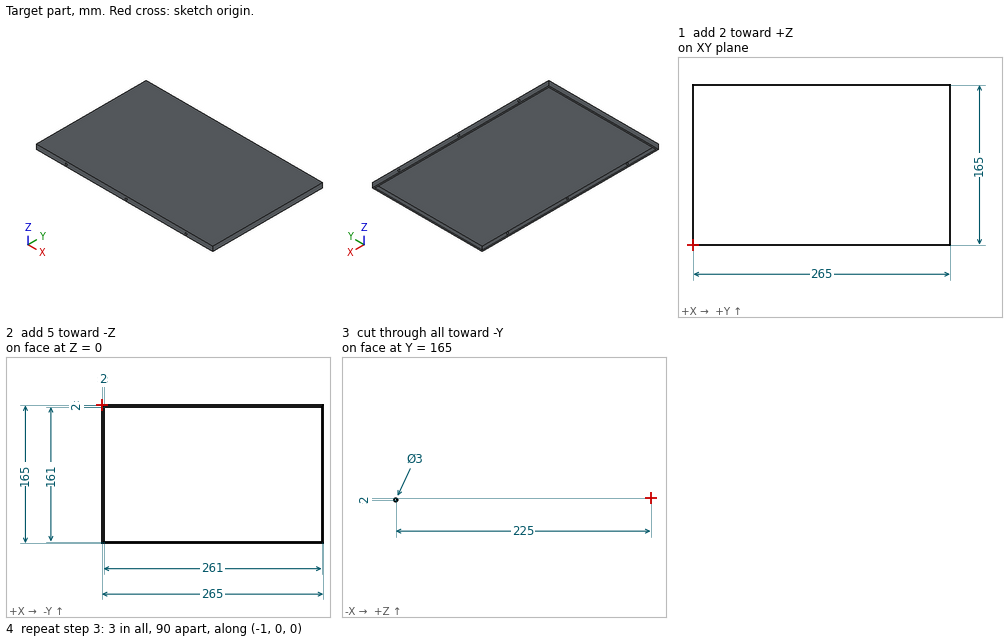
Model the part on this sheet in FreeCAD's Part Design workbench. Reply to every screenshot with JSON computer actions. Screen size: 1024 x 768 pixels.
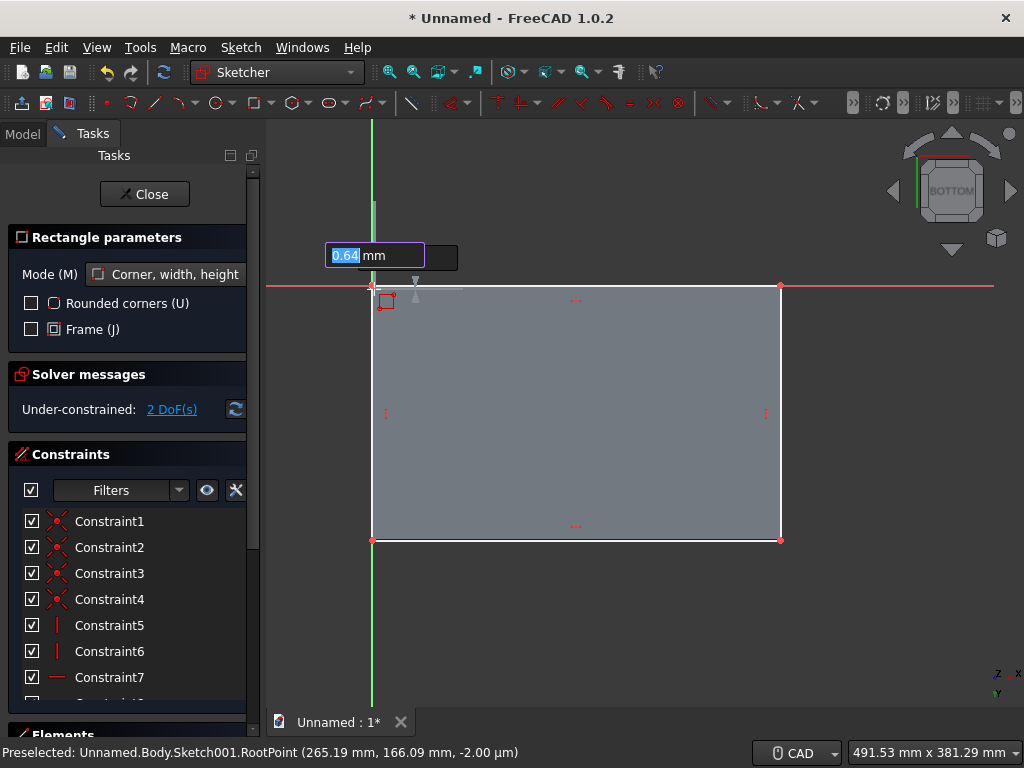
{"action": "scroll", "coordinate": [778, 537], "scroll_direction": "up", "scroll_amount": 9}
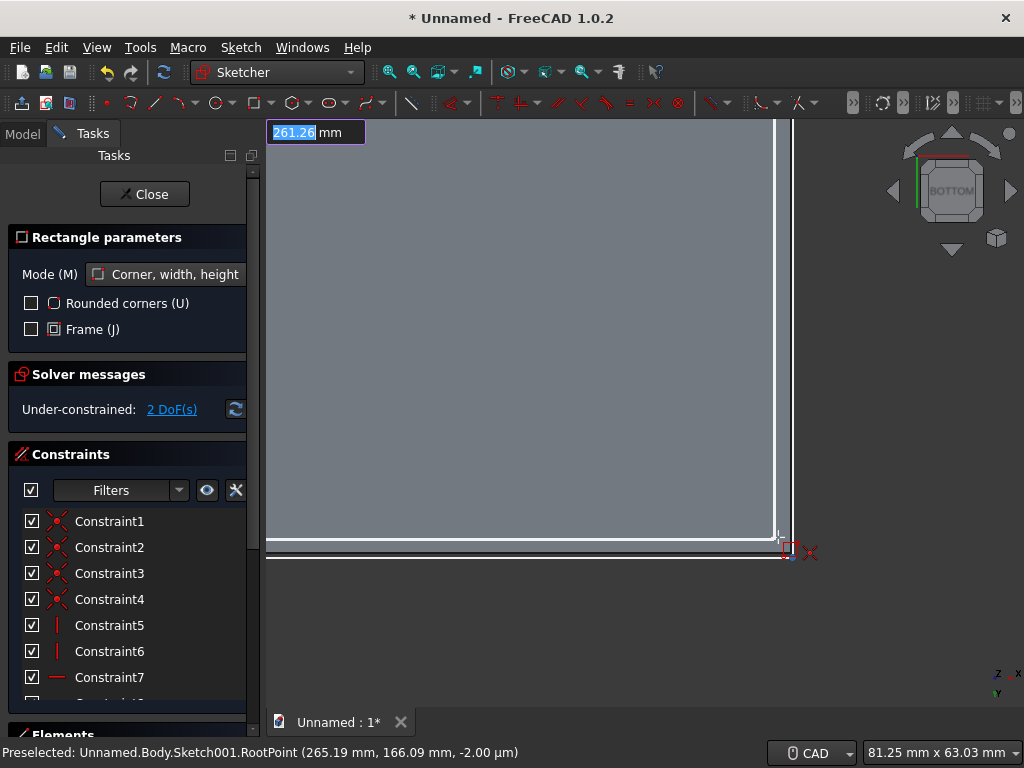
{"action": "left_click", "coordinate": [772, 535]}
{"action": "key", "text": "Escape"}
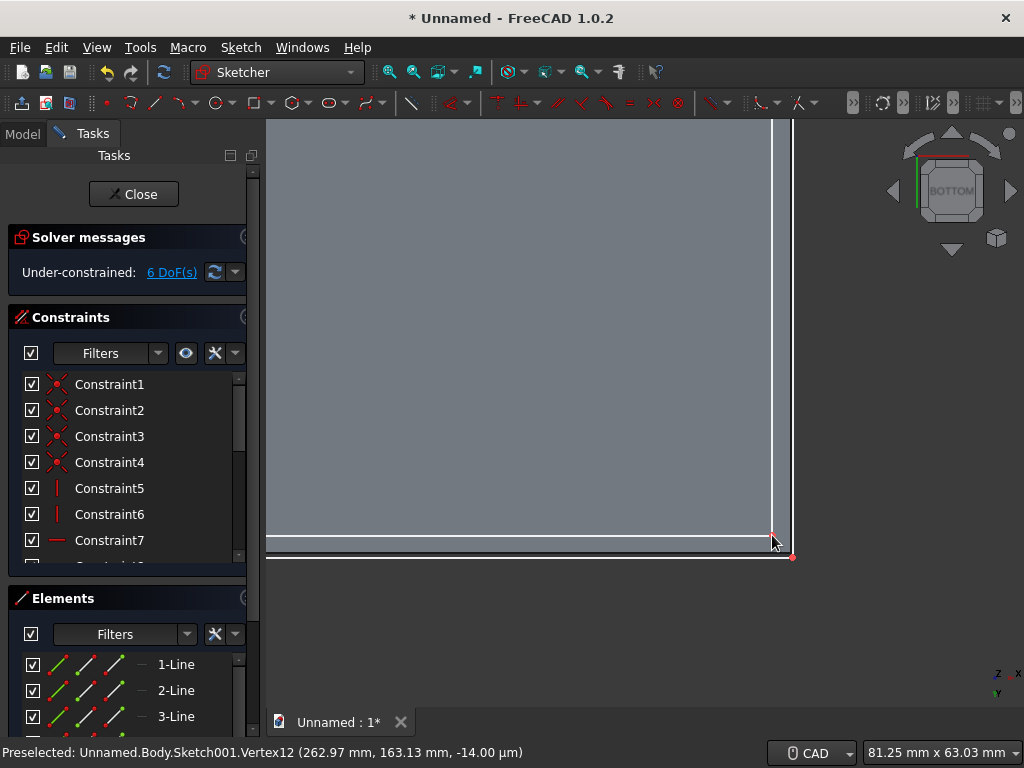
{"action": "left_click", "coordinate": [450, 104]}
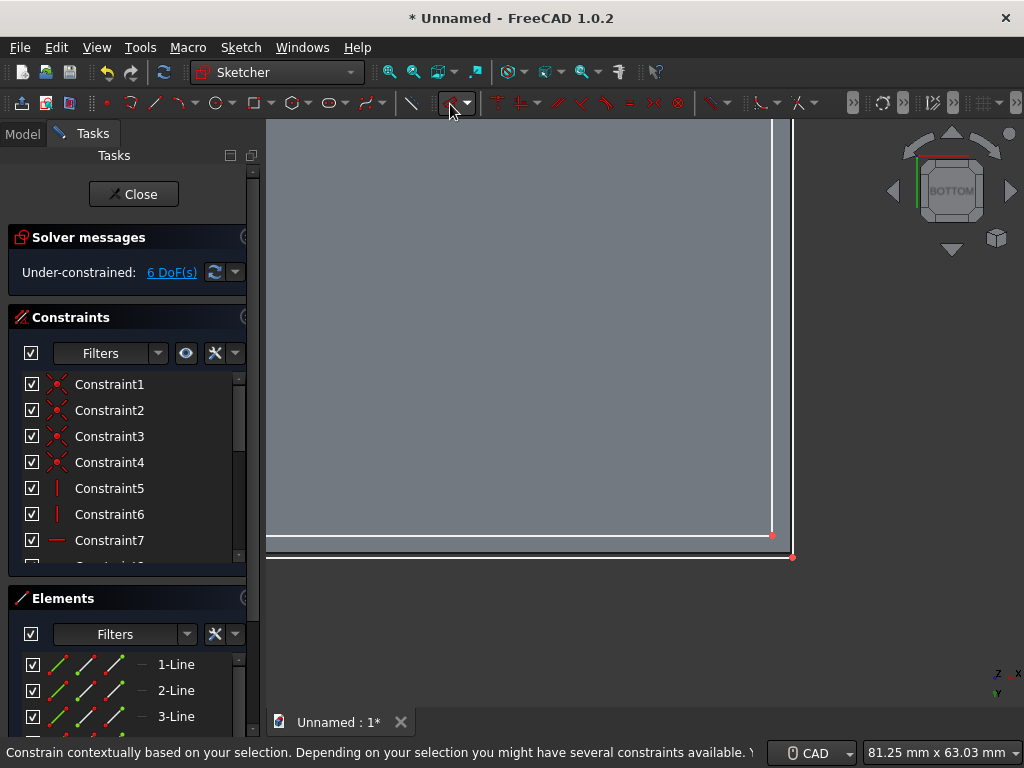
{"action": "scroll", "coordinate": [779, 538], "scroll_direction": "down", "scroll_amount": 9}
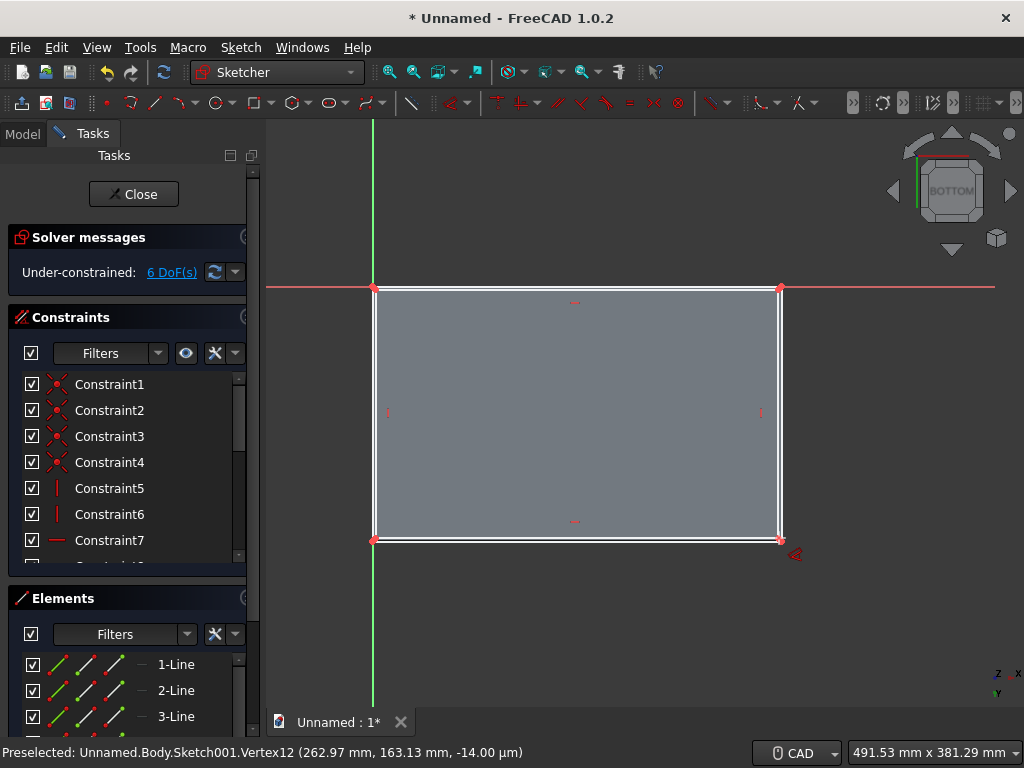
{"action": "scroll", "coordinate": [376, 290], "scroll_direction": "up", "scroll_amount": 13}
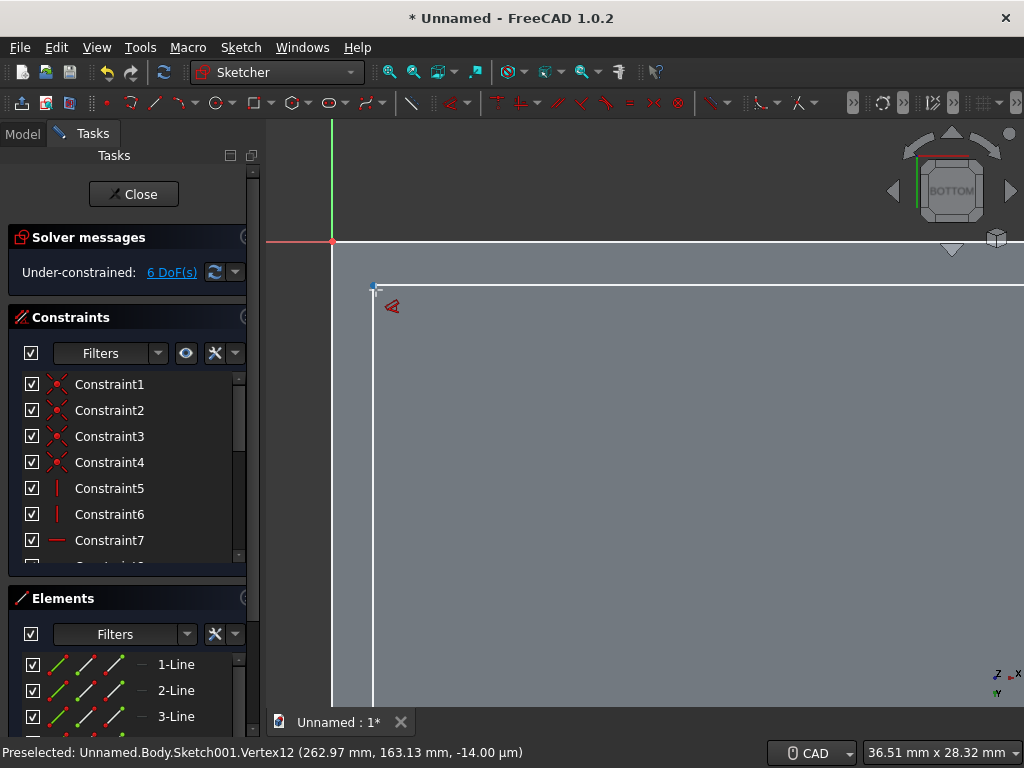
{"action": "left_click", "coordinate": [373, 285]}
{"action": "left_click", "coordinate": [353, 208]}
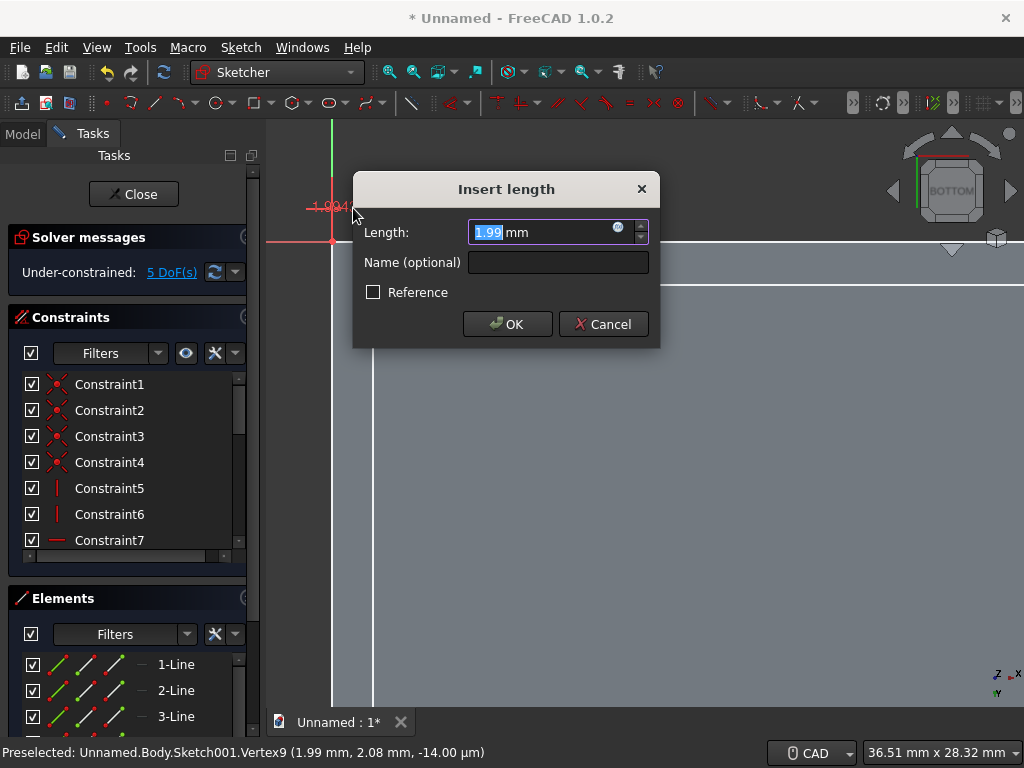
{"action": "type", "text": "2"}
{"action": "key", "text": "Return"}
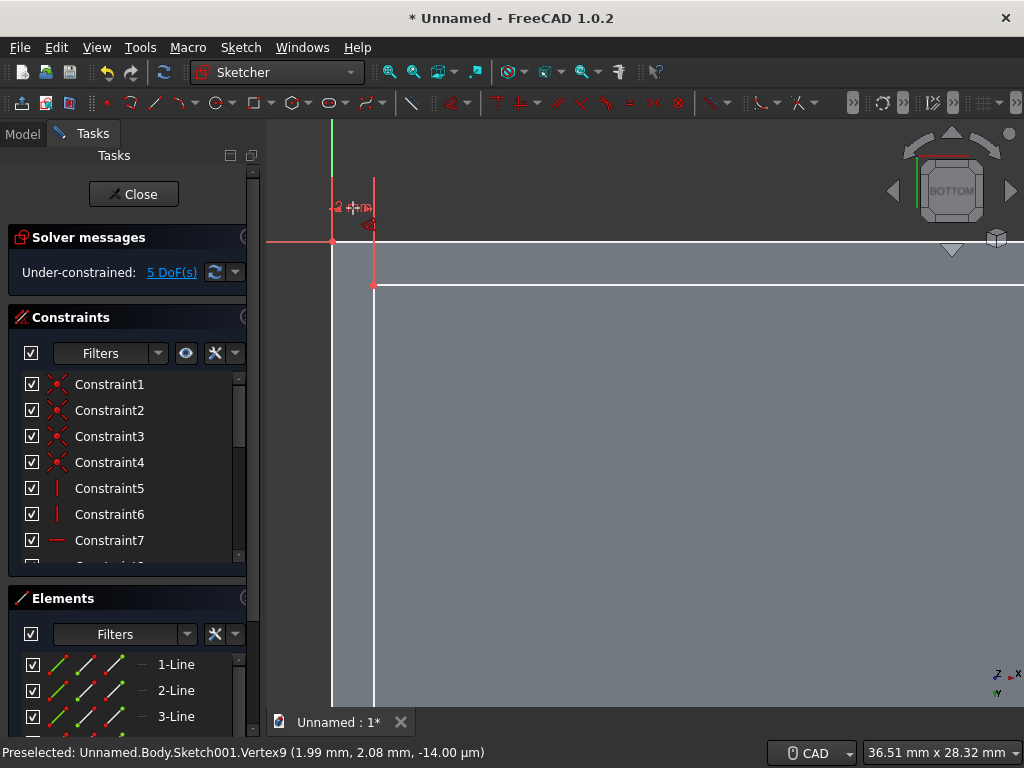
{"action": "left_click", "coordinate": [374, 285]}
{"action": "left_click", "coordinate": [298, 264]}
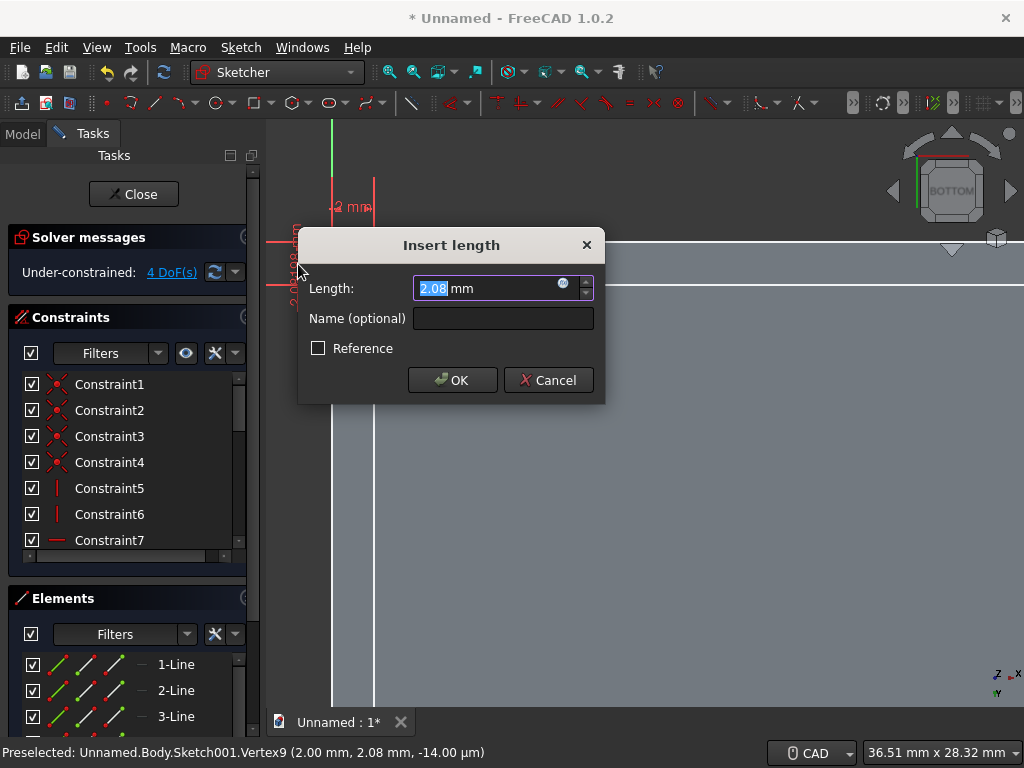
{"action": "type", "text": "2"}
{"action": "key", "text": "Return"}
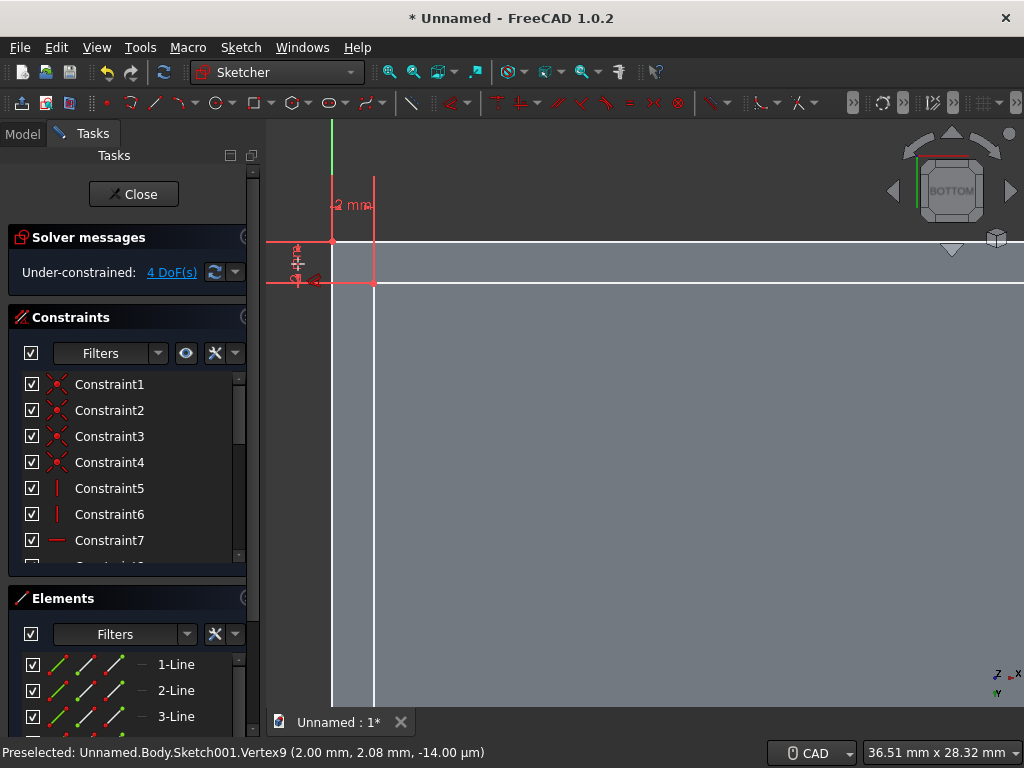
{"action": "scroll", "coordinate": [375, 289], "scroll_direction": "down", "scroll_amount": 13}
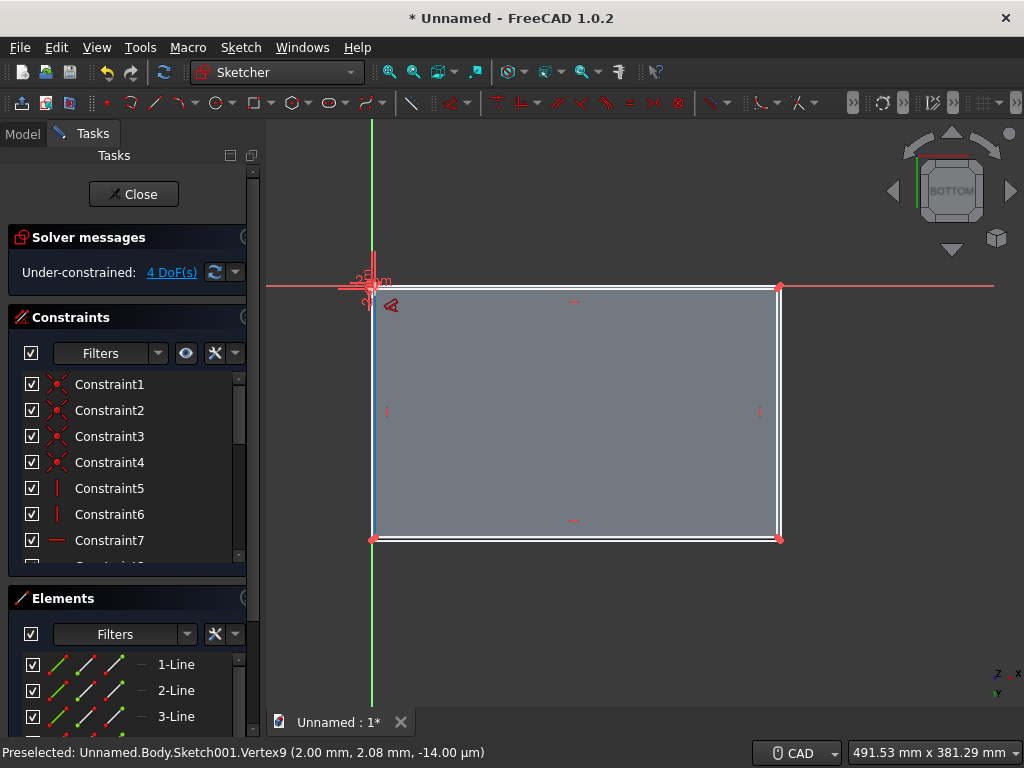
{"action": "scroll", "coordinate": [372, 362], "scroll_direction": "up", "scroll_amount": 8}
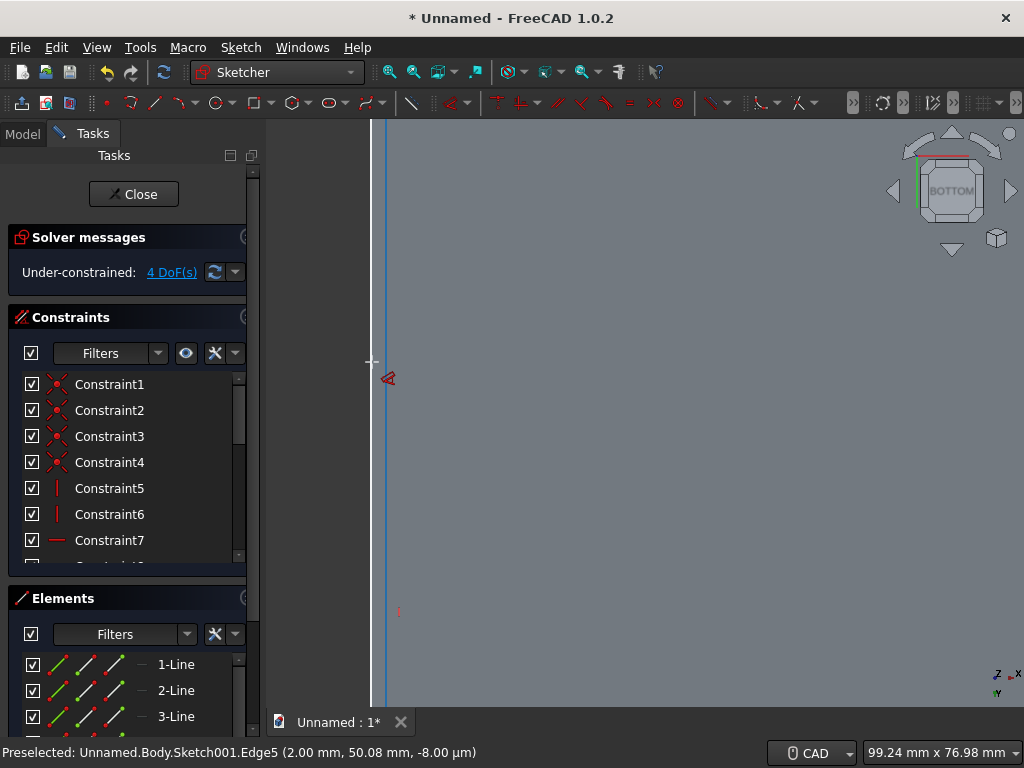
{"action": "left_click", "coordinate": [371, 362]}
{"action": "left_click", "coordinate": [337, 413]}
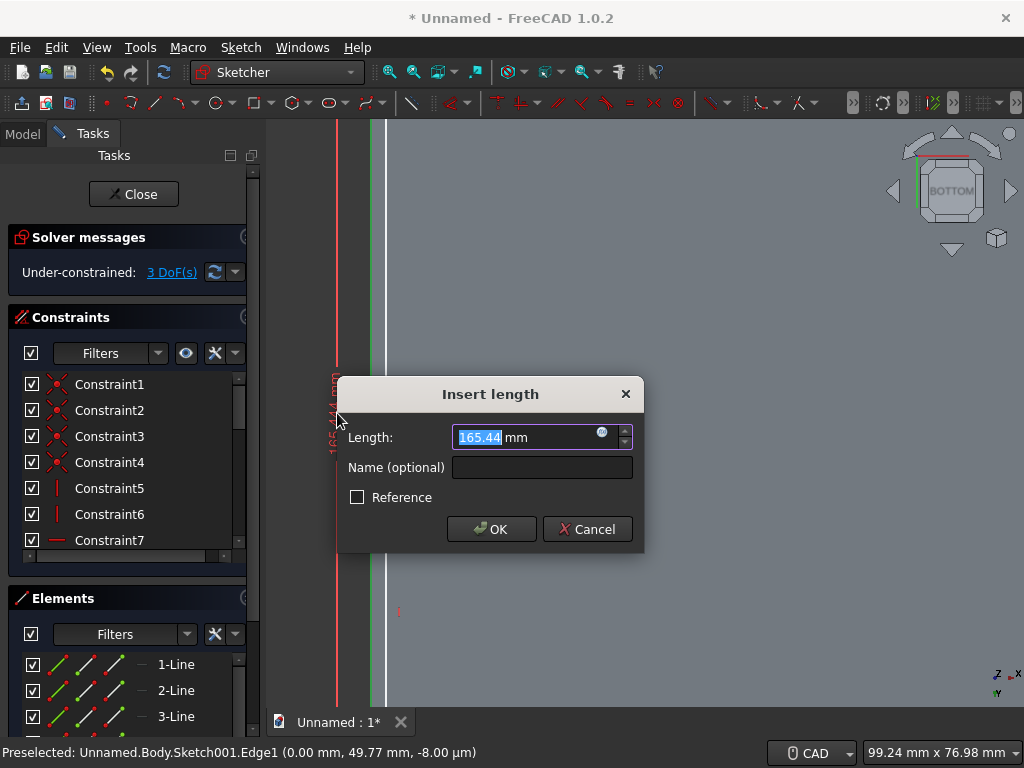
{"action": "type", "text": "165"}
{"action": "key", "text": "Return"}